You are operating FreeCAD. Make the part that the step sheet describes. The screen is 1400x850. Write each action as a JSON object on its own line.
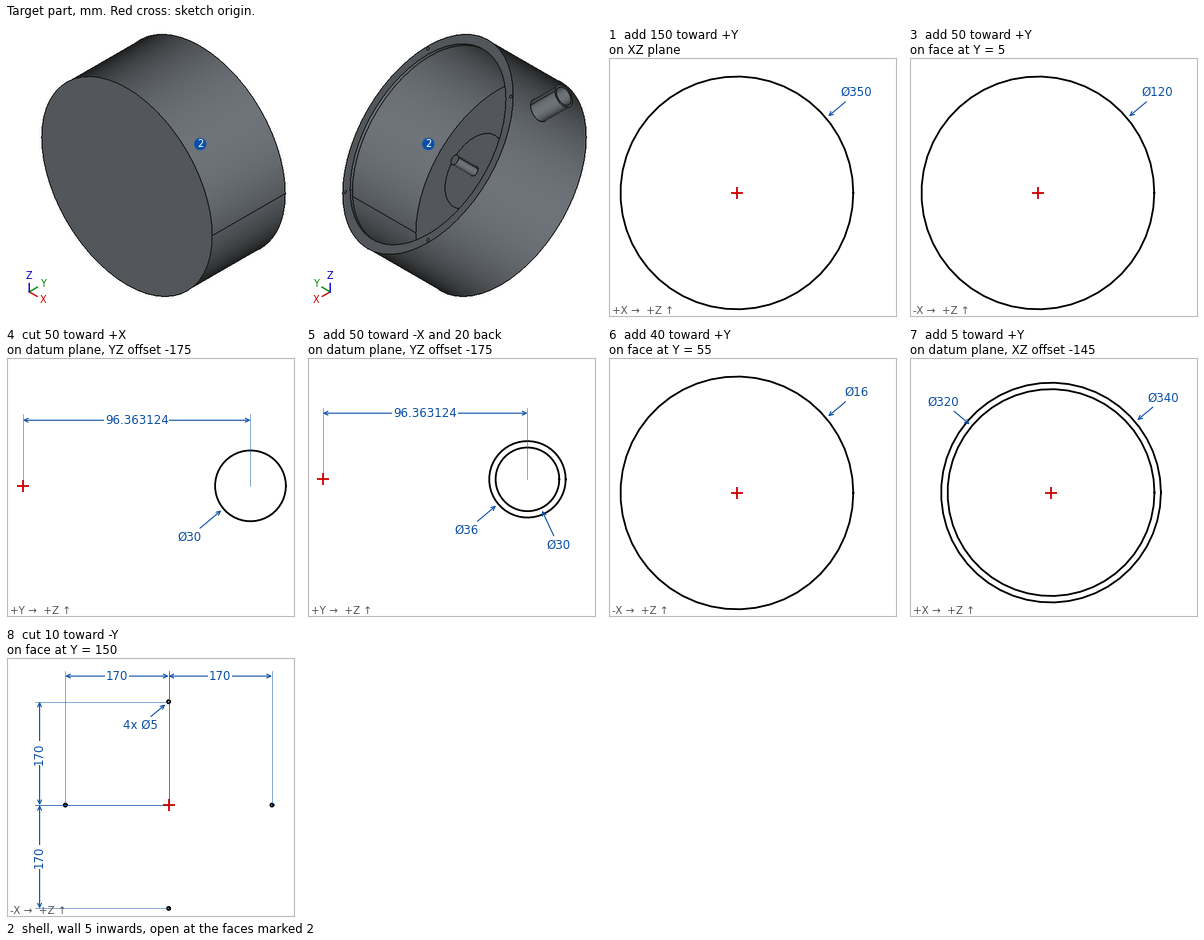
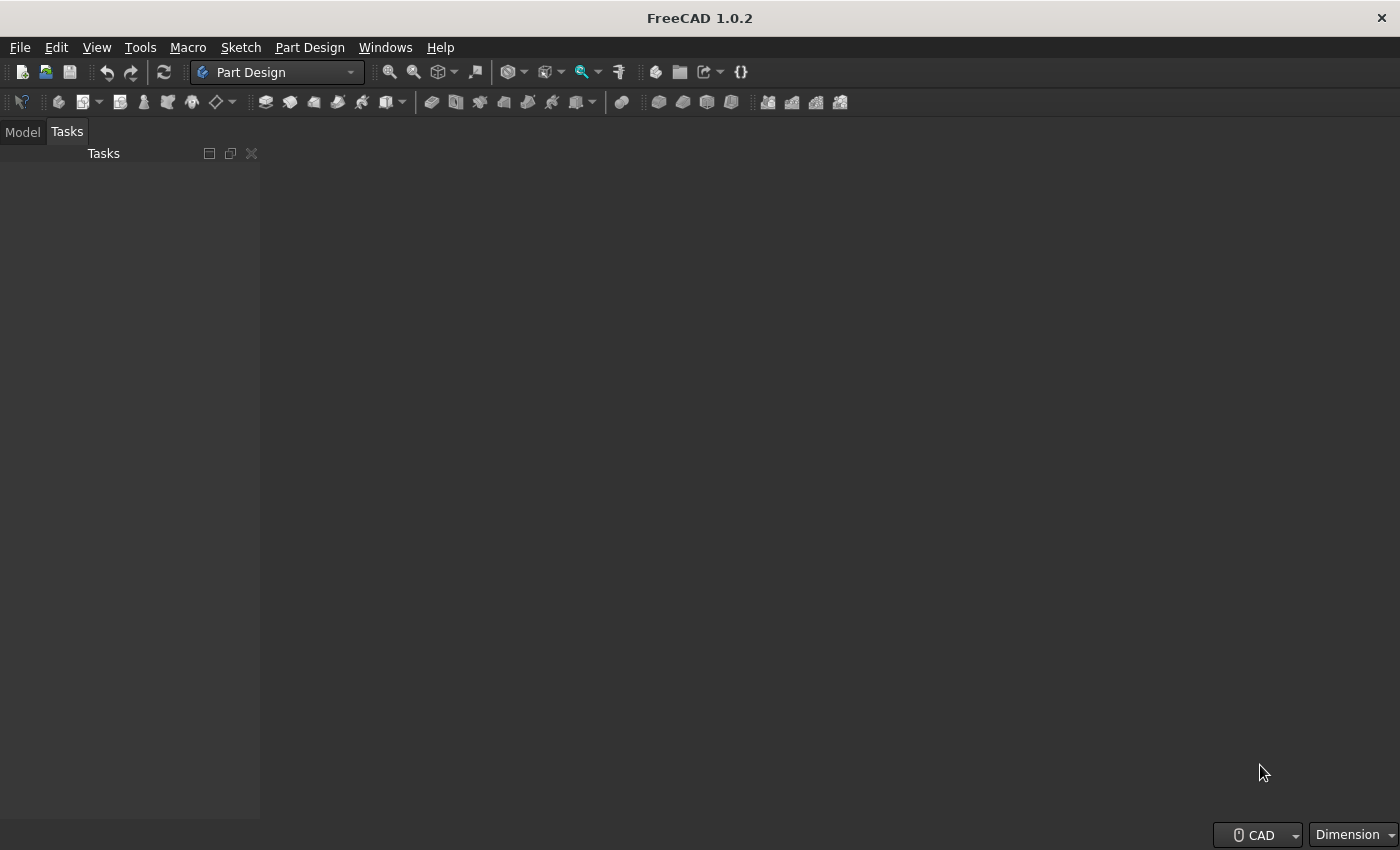
{"action": "left_click", "coordinate": [1126, 72]}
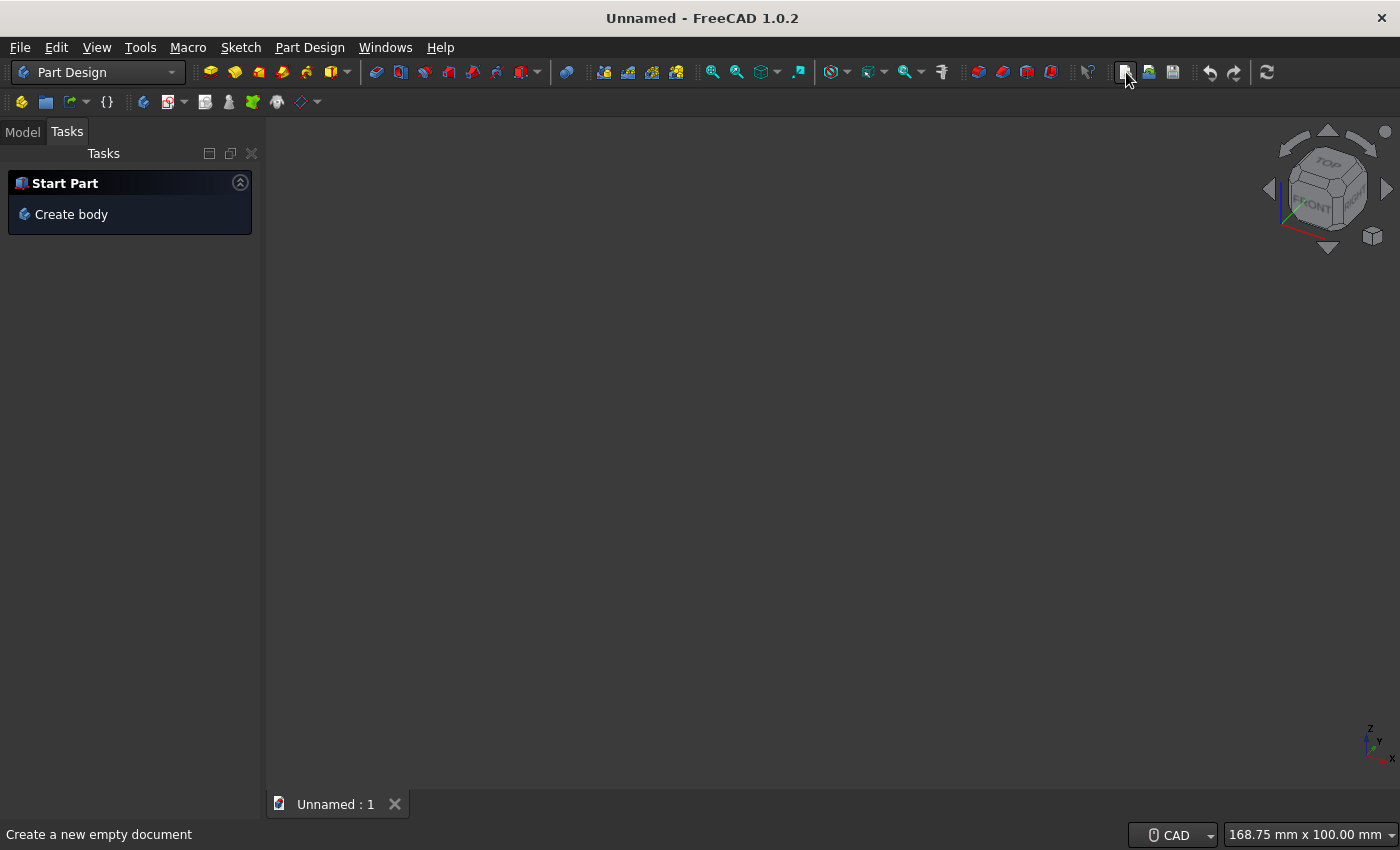
{"action": "left_click", "coordinate": [168, 102]}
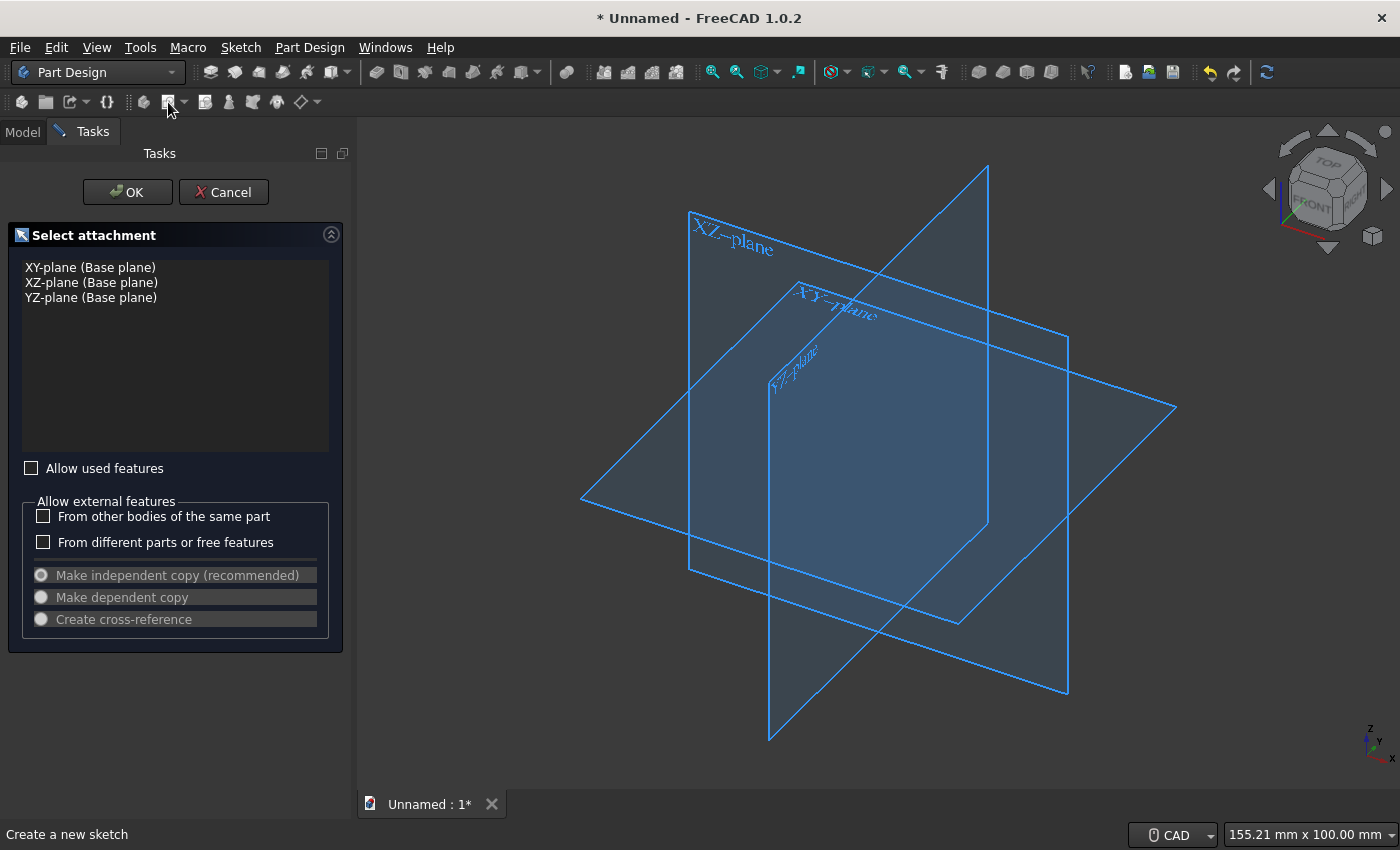
{"action": "left_click", "coordinate": [82, 282]}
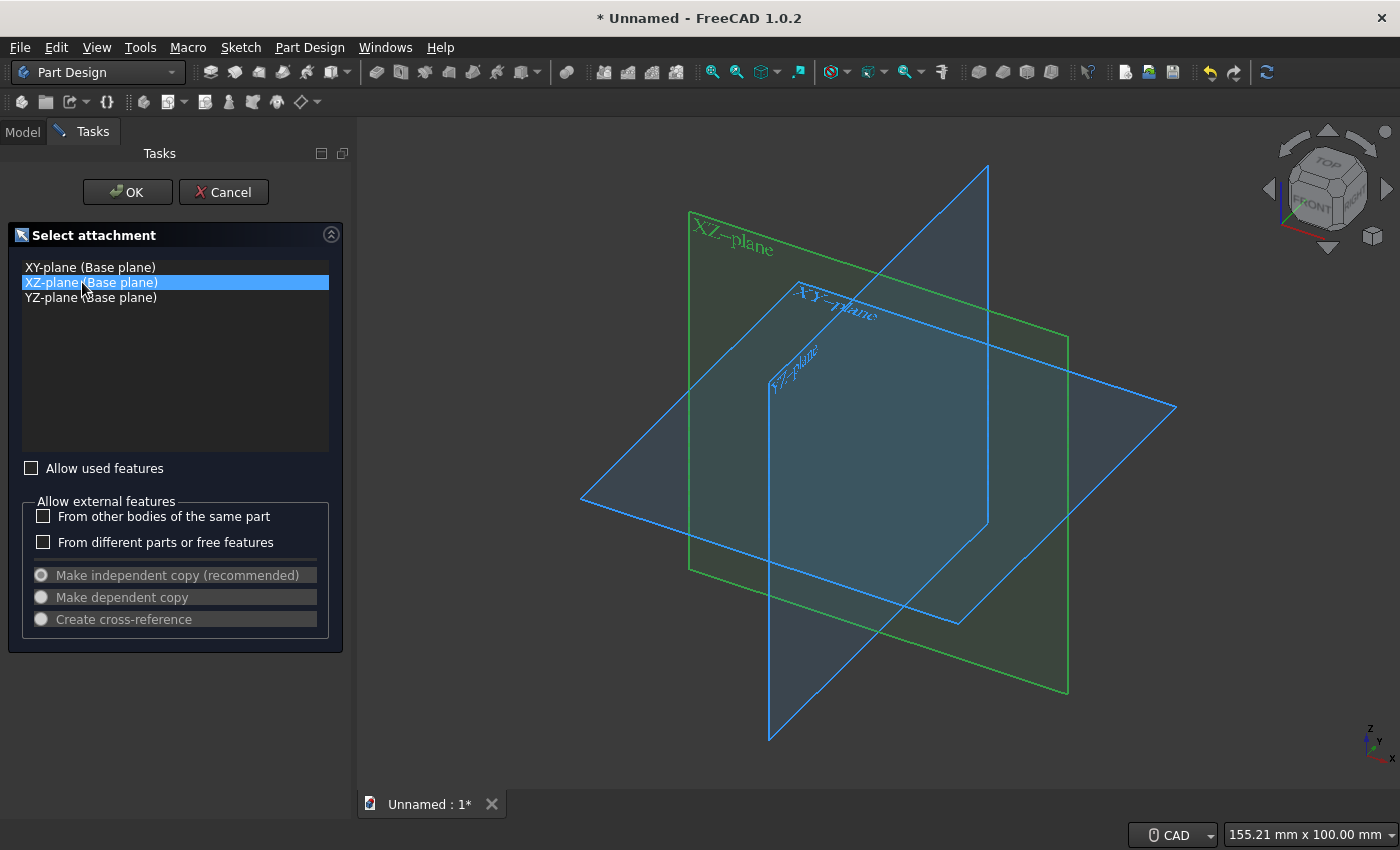
{"action": "left_click", "coordinate": [128, 192]}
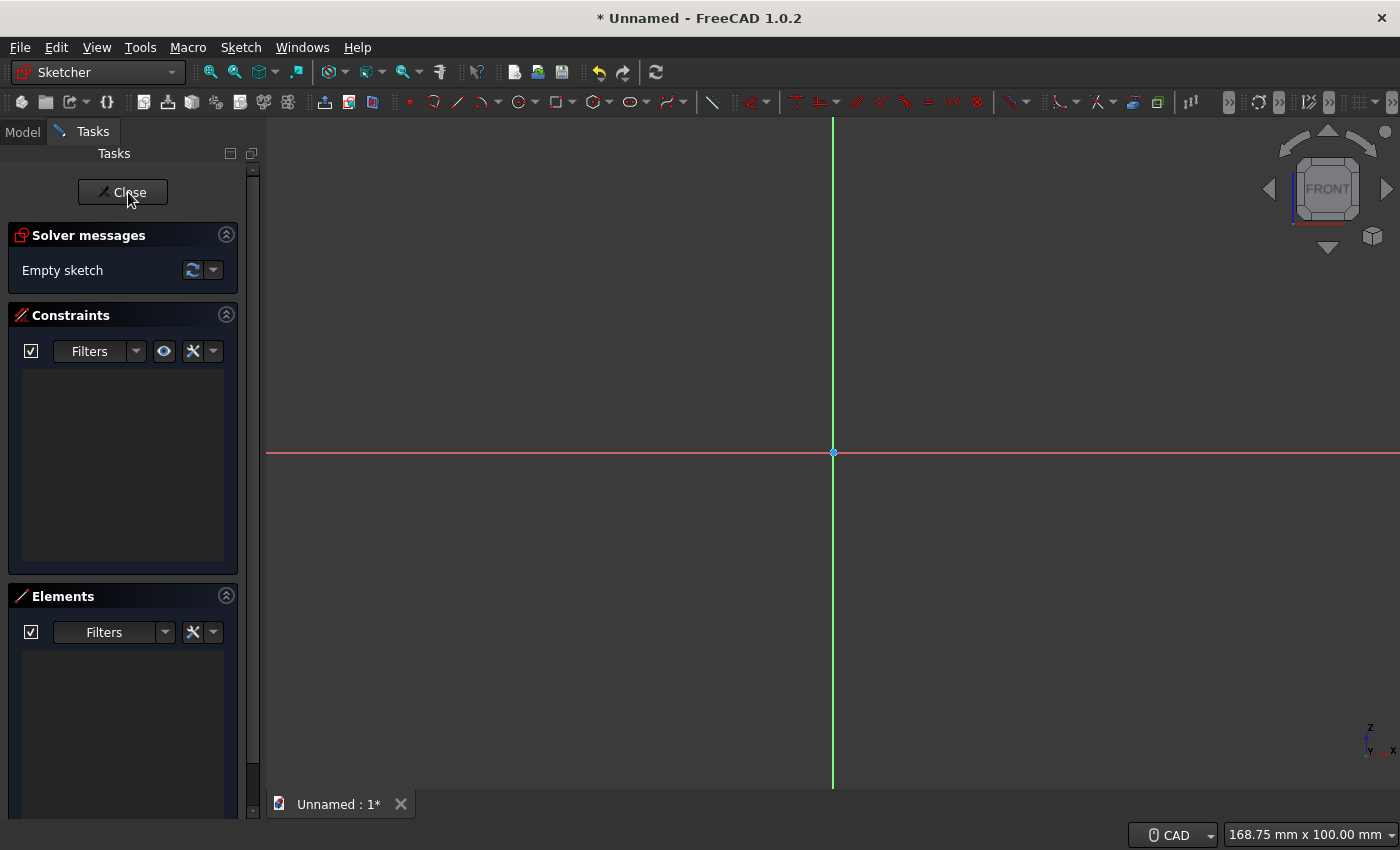
{"action": "scroll", "coordinate": [747, 453], "scroll_direction": "down", "scroll_amount": 8}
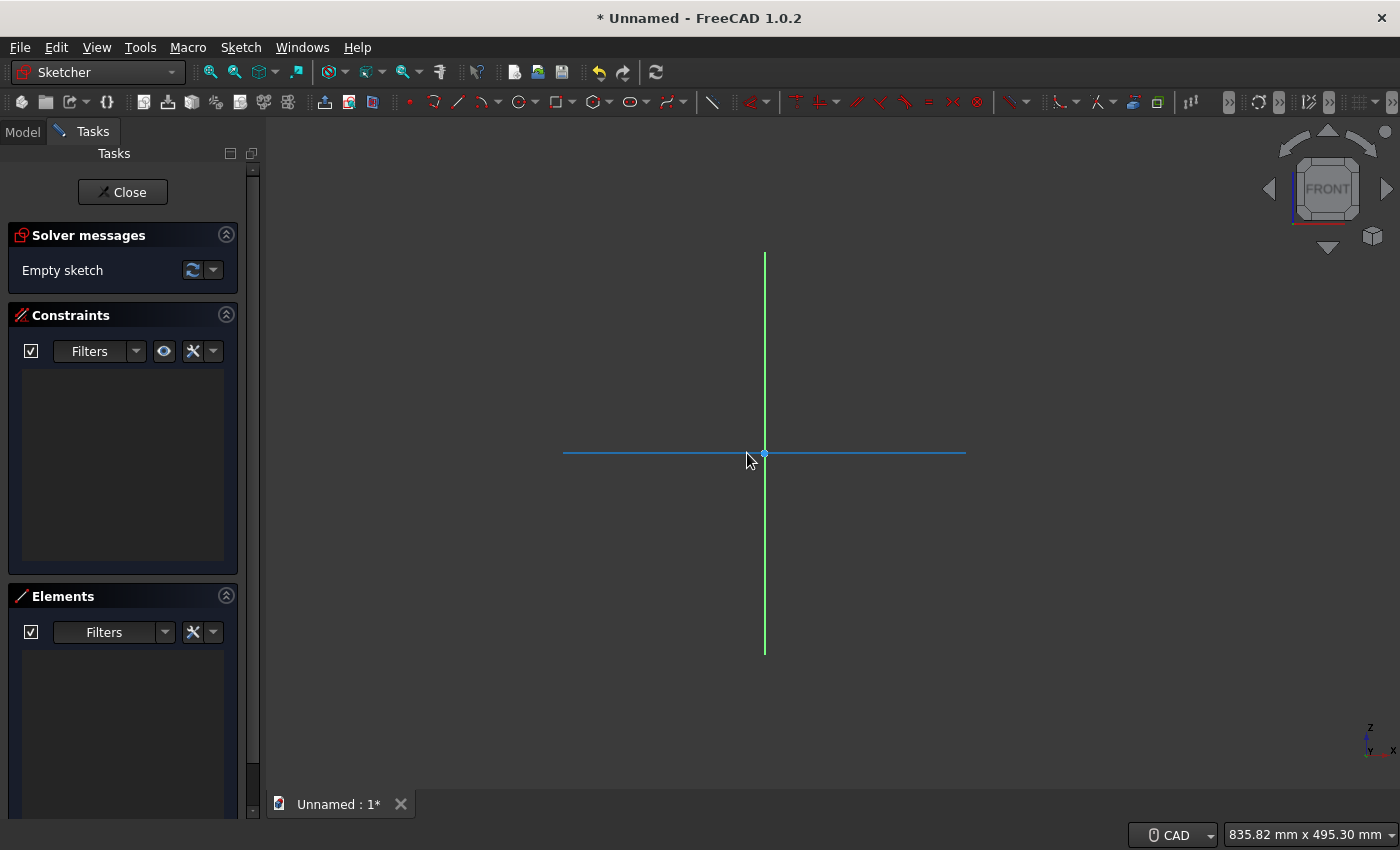
{"action": "left_click", "coordinate": [520, 102]}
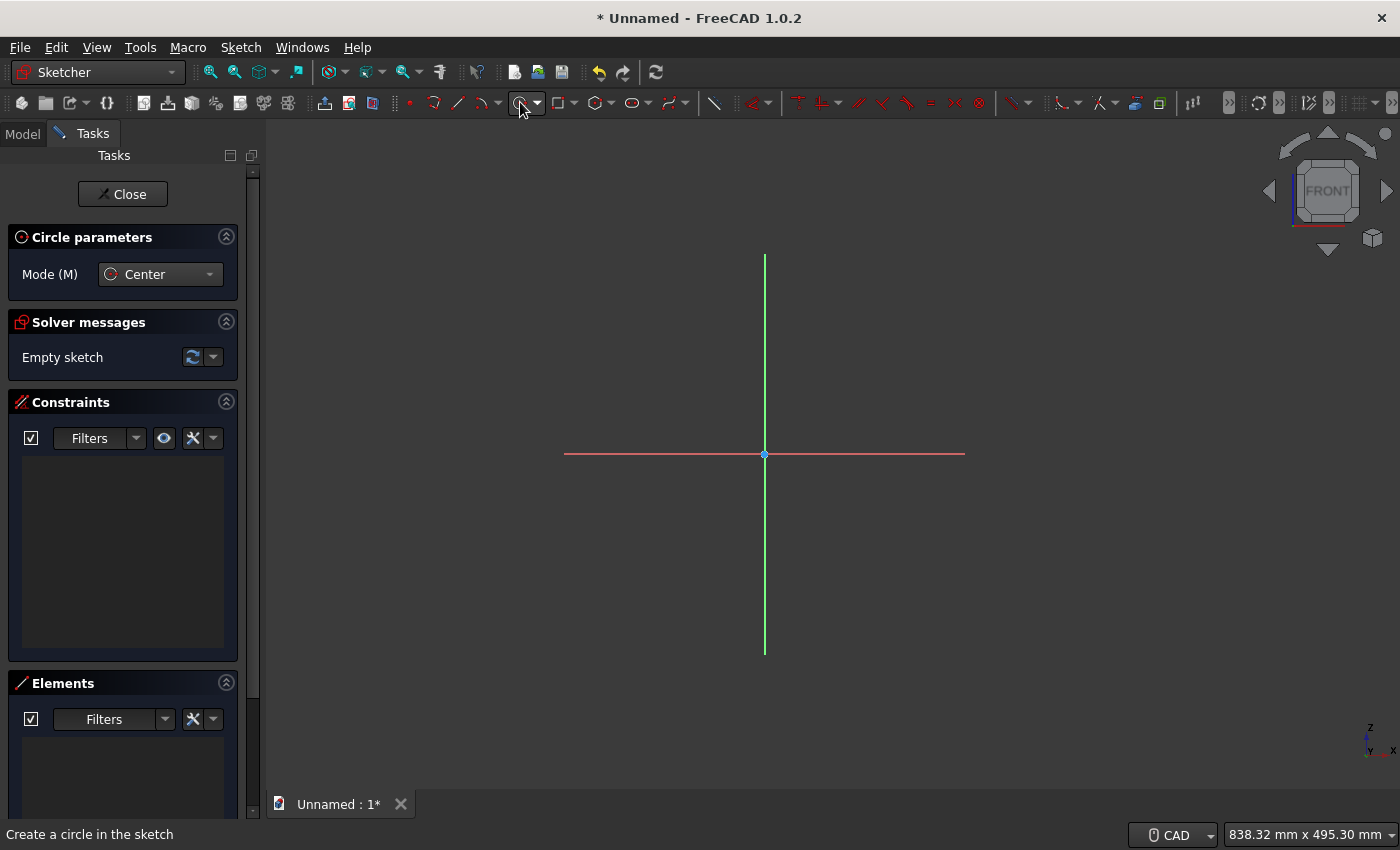
{"action": "left_click", "coordinate": [765, 454]}
{"action": "mouse_move", "coordinate": [932, 287]}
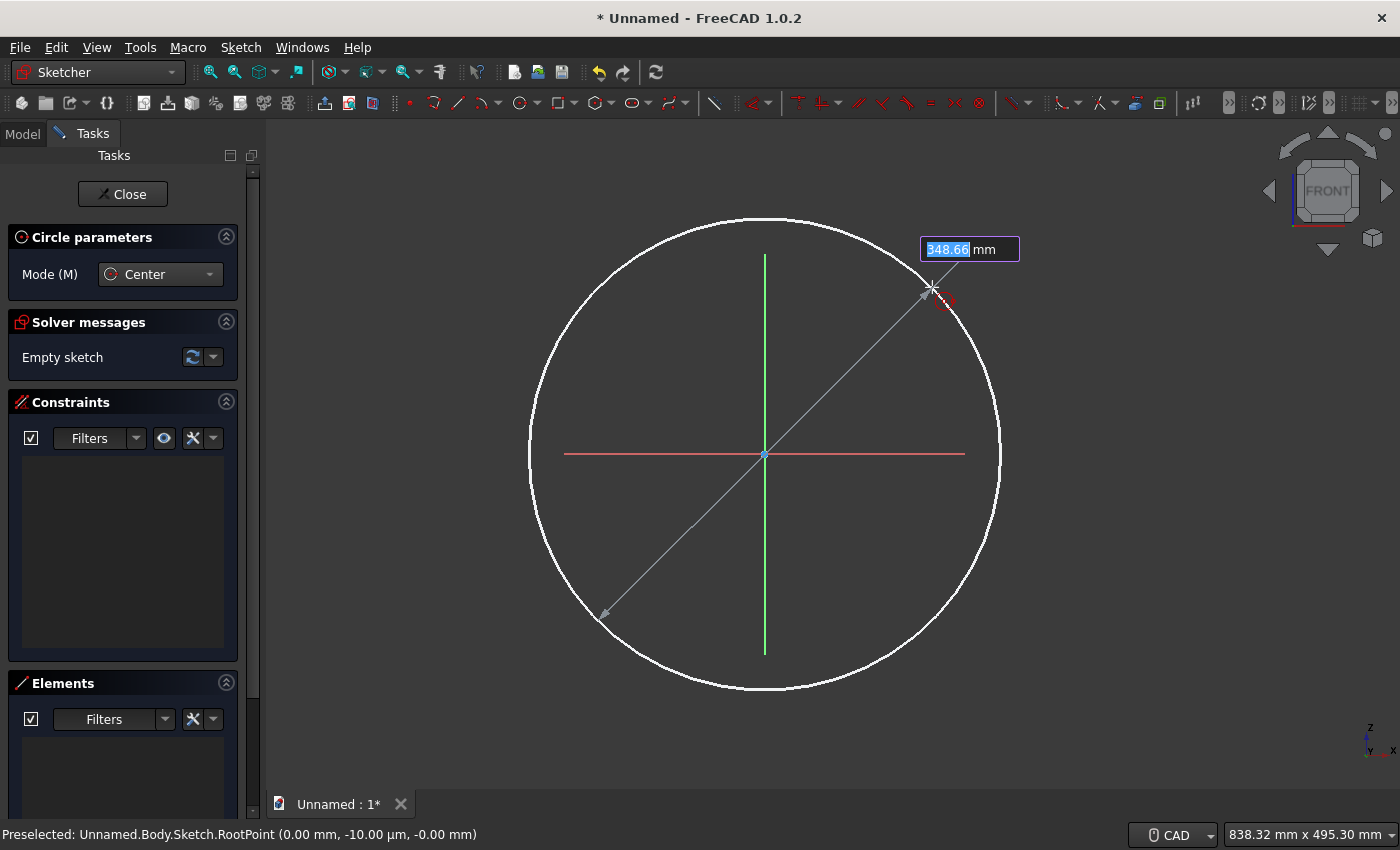
{"action": "type", "text": "350"}
{"action": "key", "text": "Return"}
{"action": "key", "text": "Escape"}